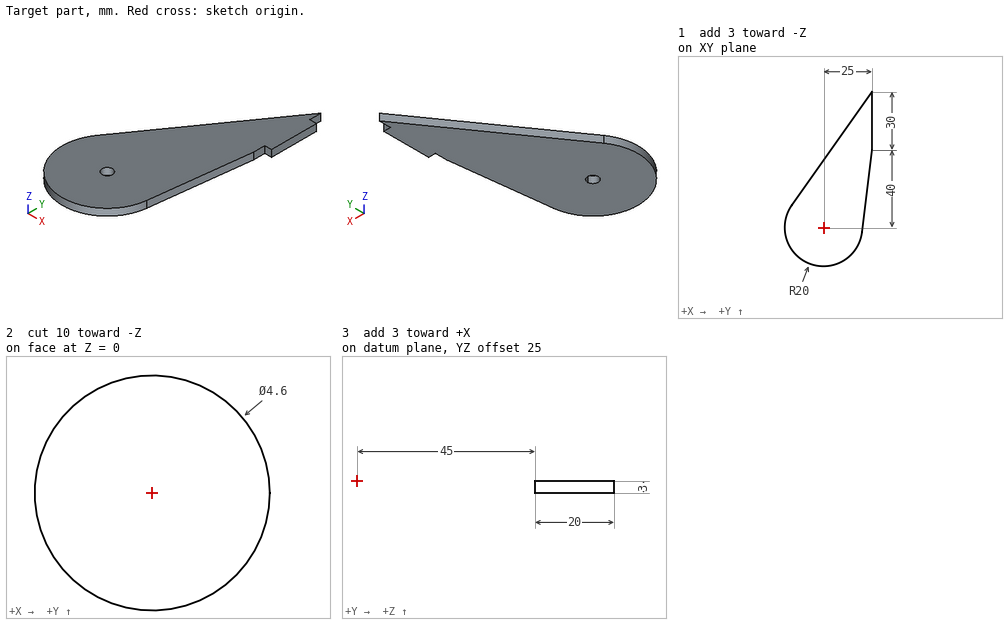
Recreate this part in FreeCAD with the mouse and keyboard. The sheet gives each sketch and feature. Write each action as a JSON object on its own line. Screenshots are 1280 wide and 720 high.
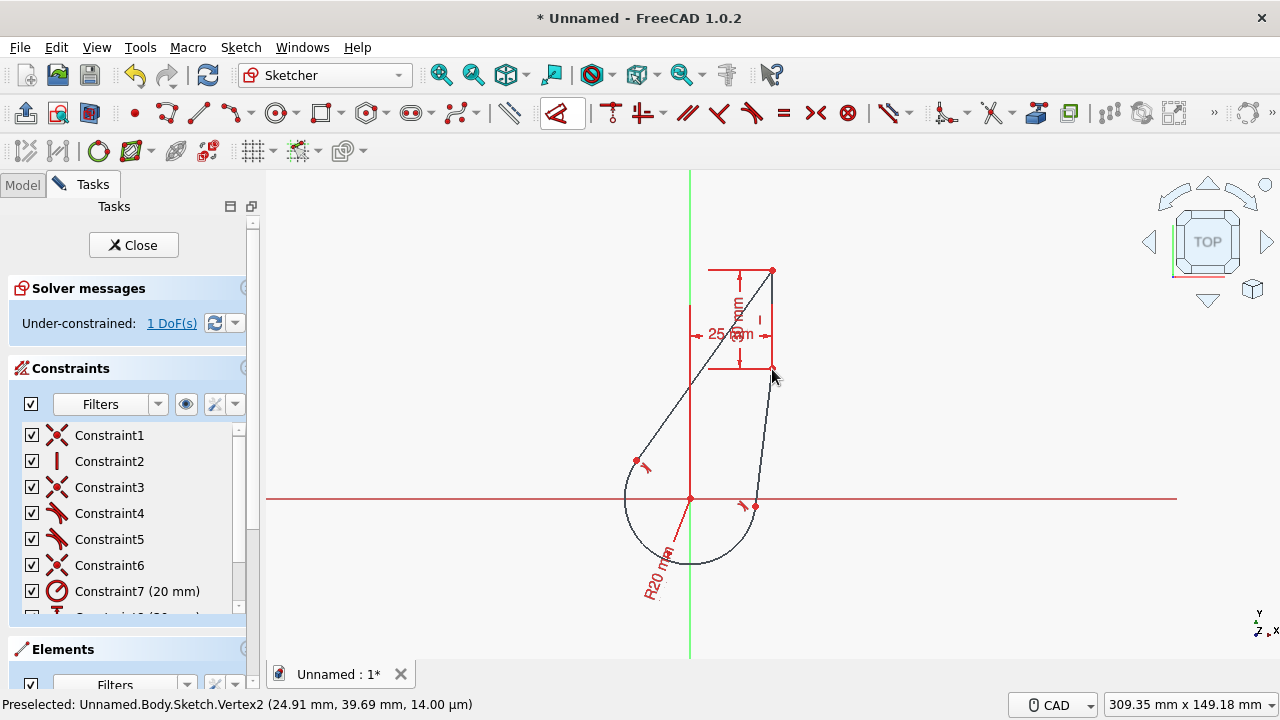
{"action": "left_click", "coordinate": [772, 369]}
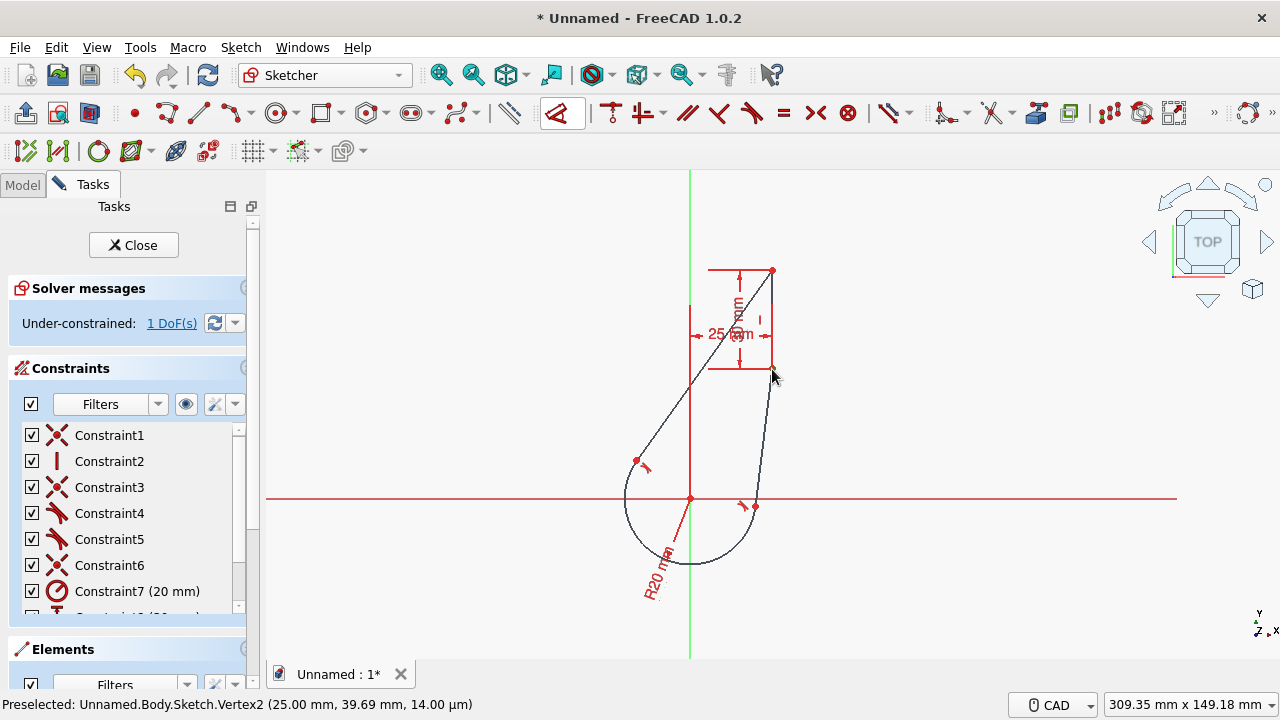
{"action": "key", "text": "i"}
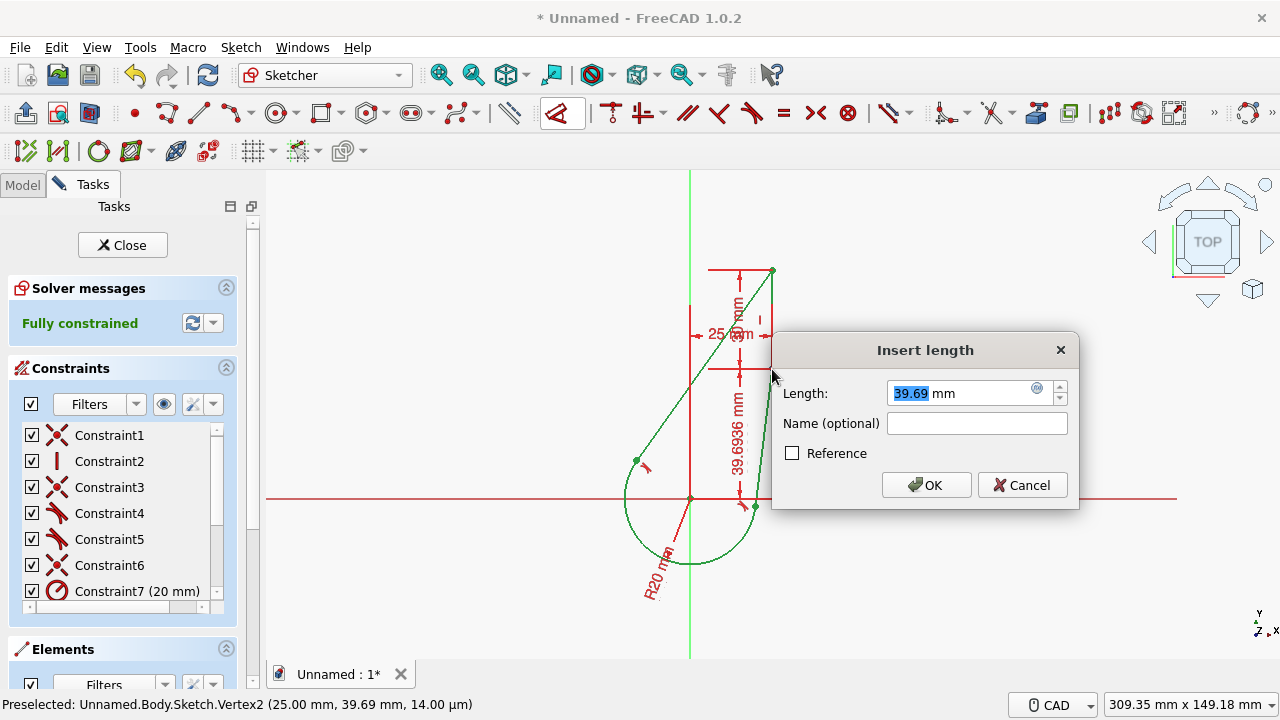
{"action": "type", "text": "40"}
{"action": "key", "text": "Return"}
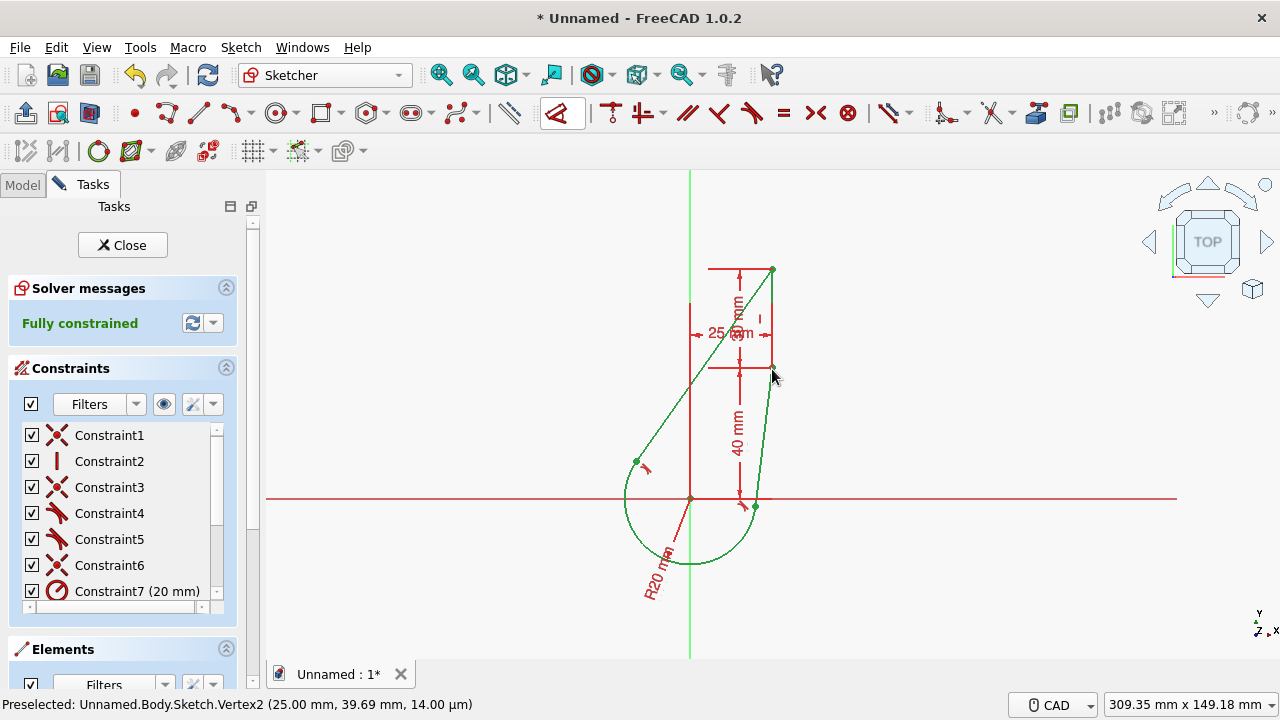
{"action": "left_click", "coordinate": [123, 245]}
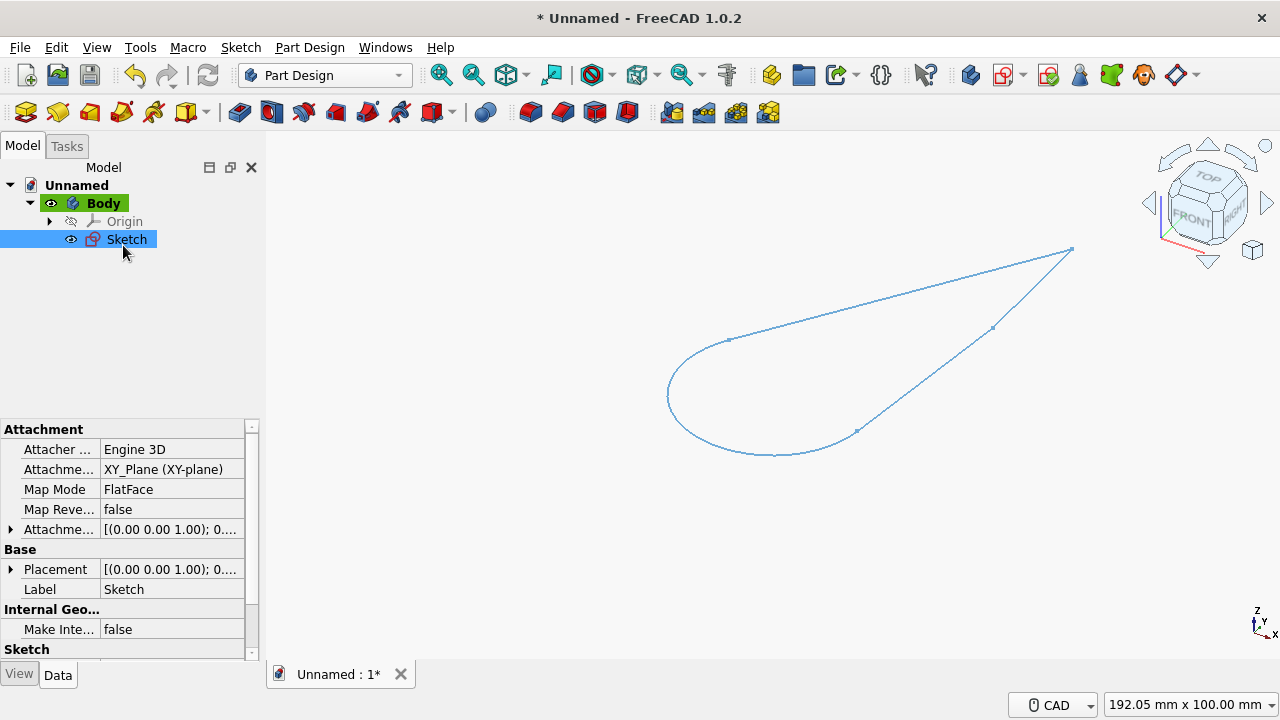
{"action": "left_click", "coordinate": [26, 112]}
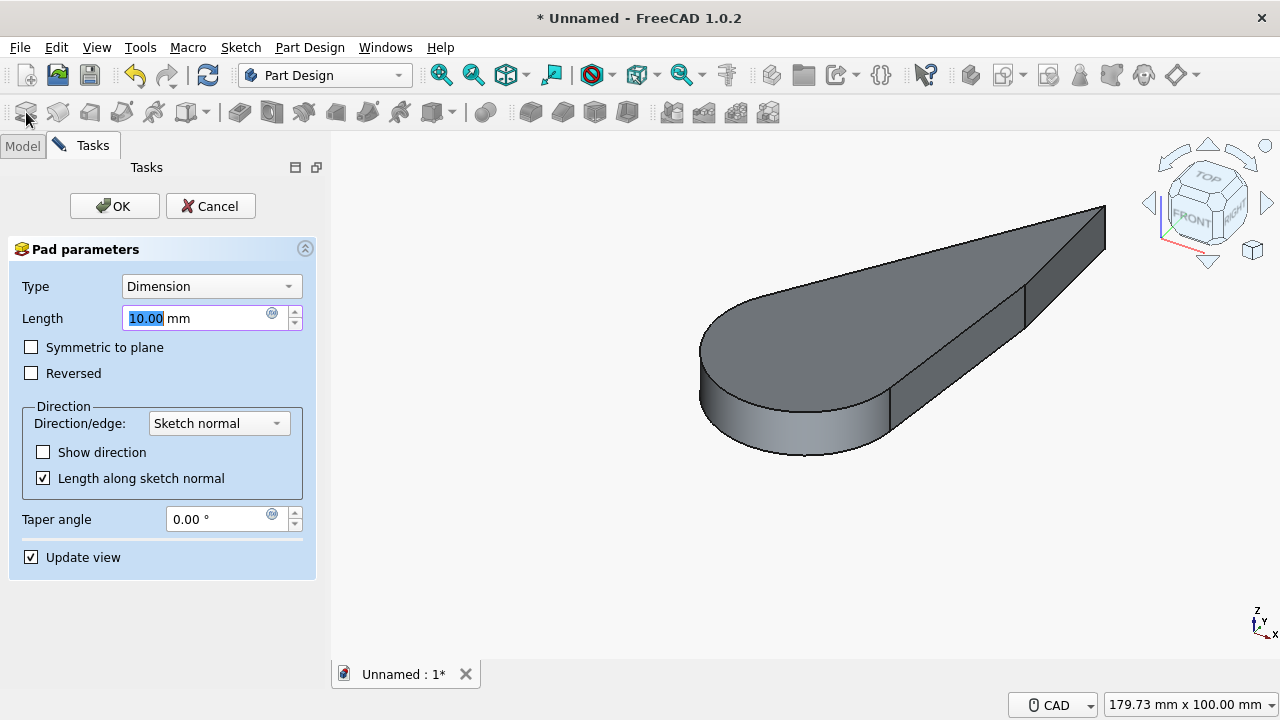
{"action": "type", "text": "3"}
{"action": "key", "text": "Tab"}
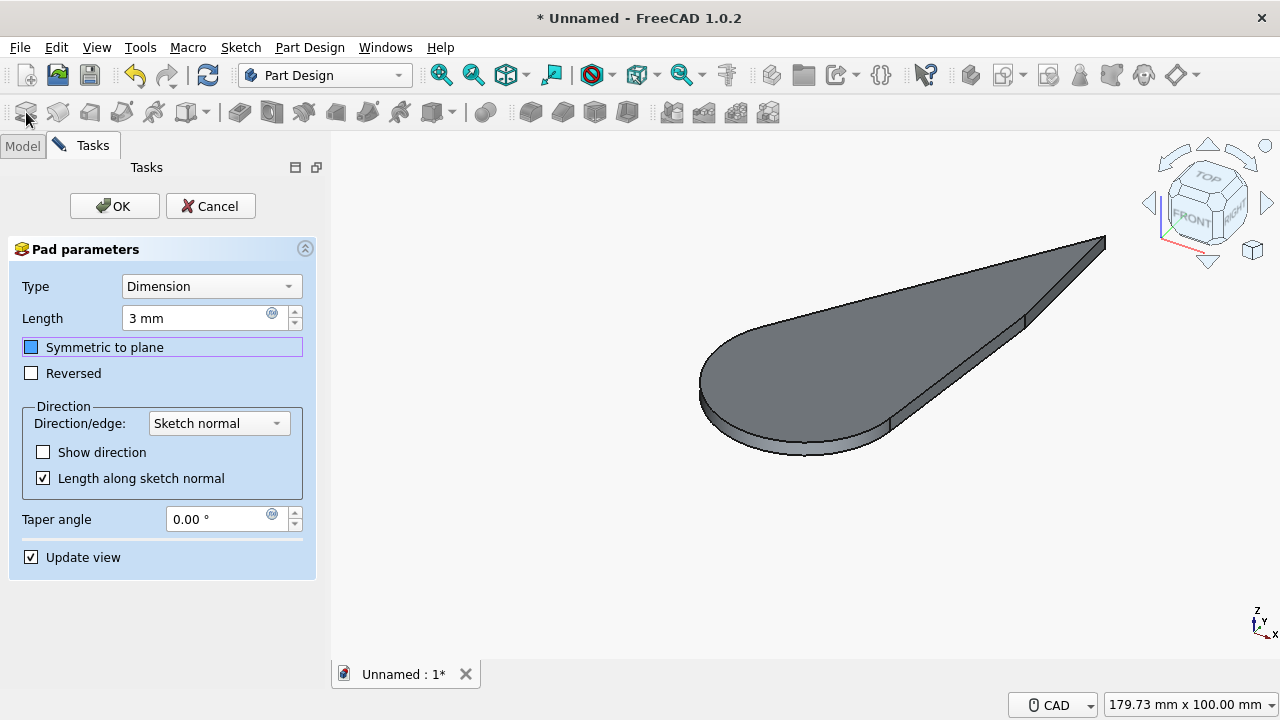
{"action": "left_click", "coordinate": [30, 373]}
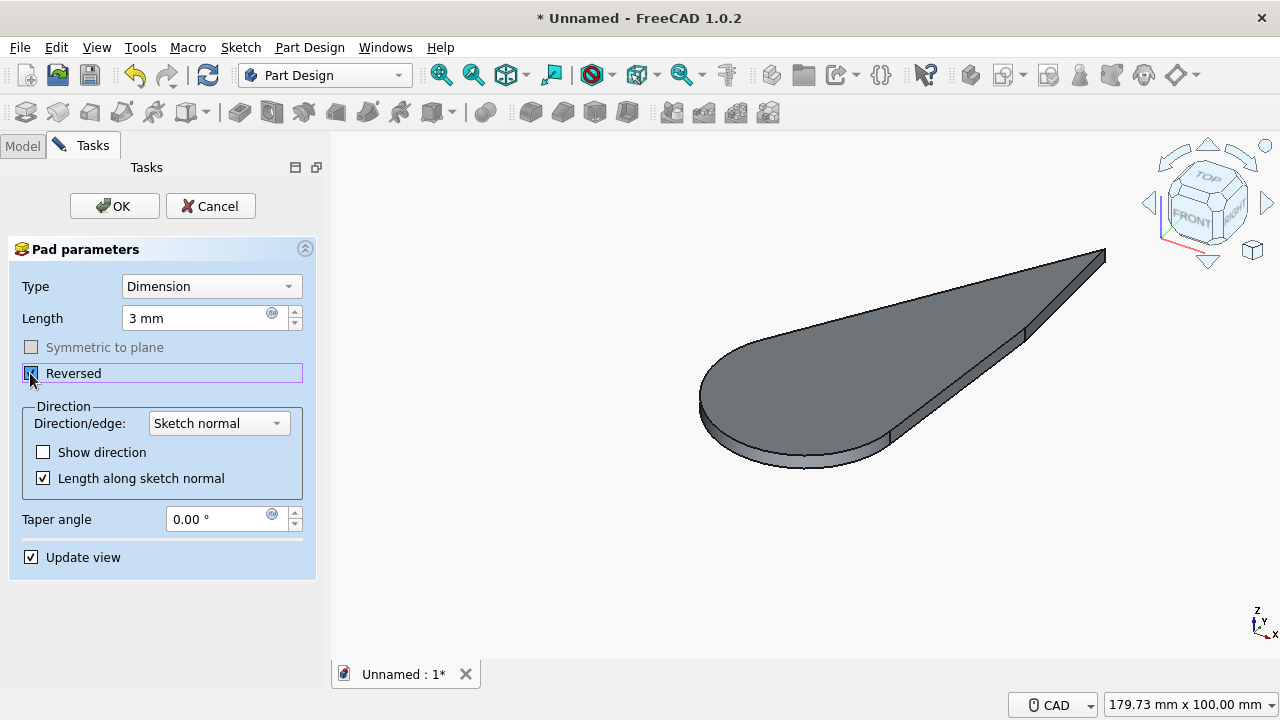
{"action": "left_click", "coordinate": [115, 206]}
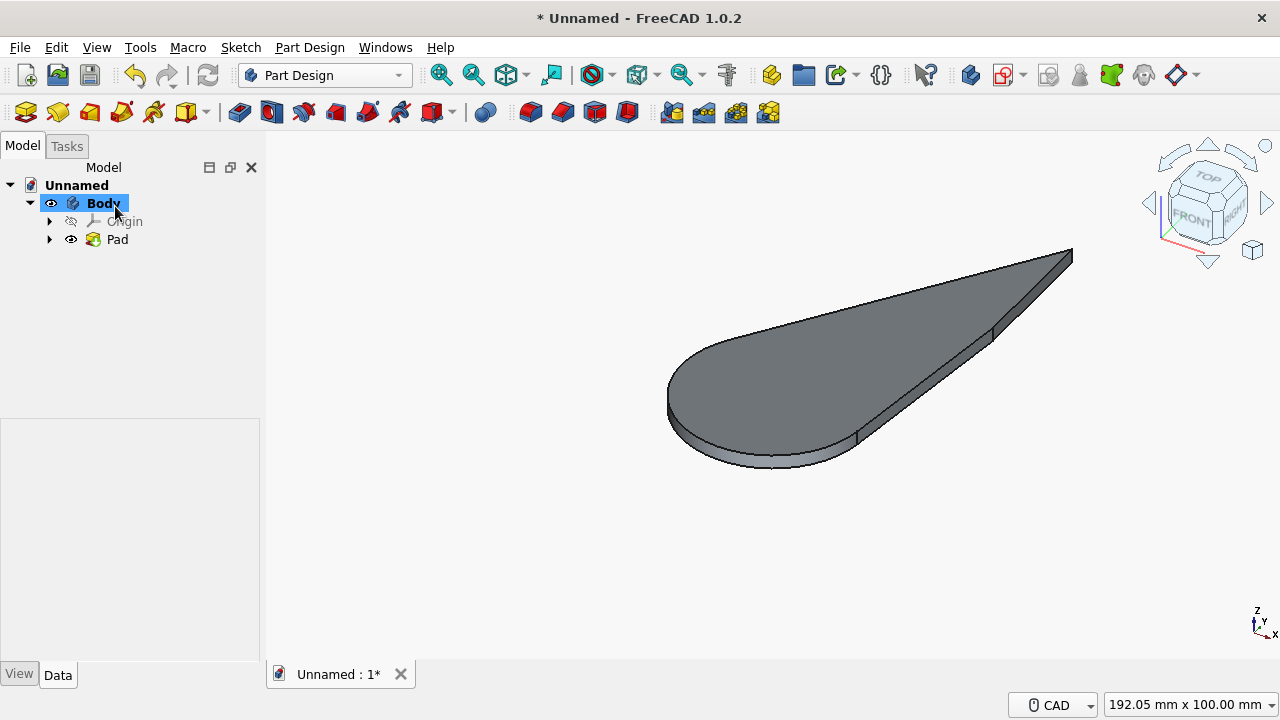
{"action": "left_click", "coordinate": [783, 400]}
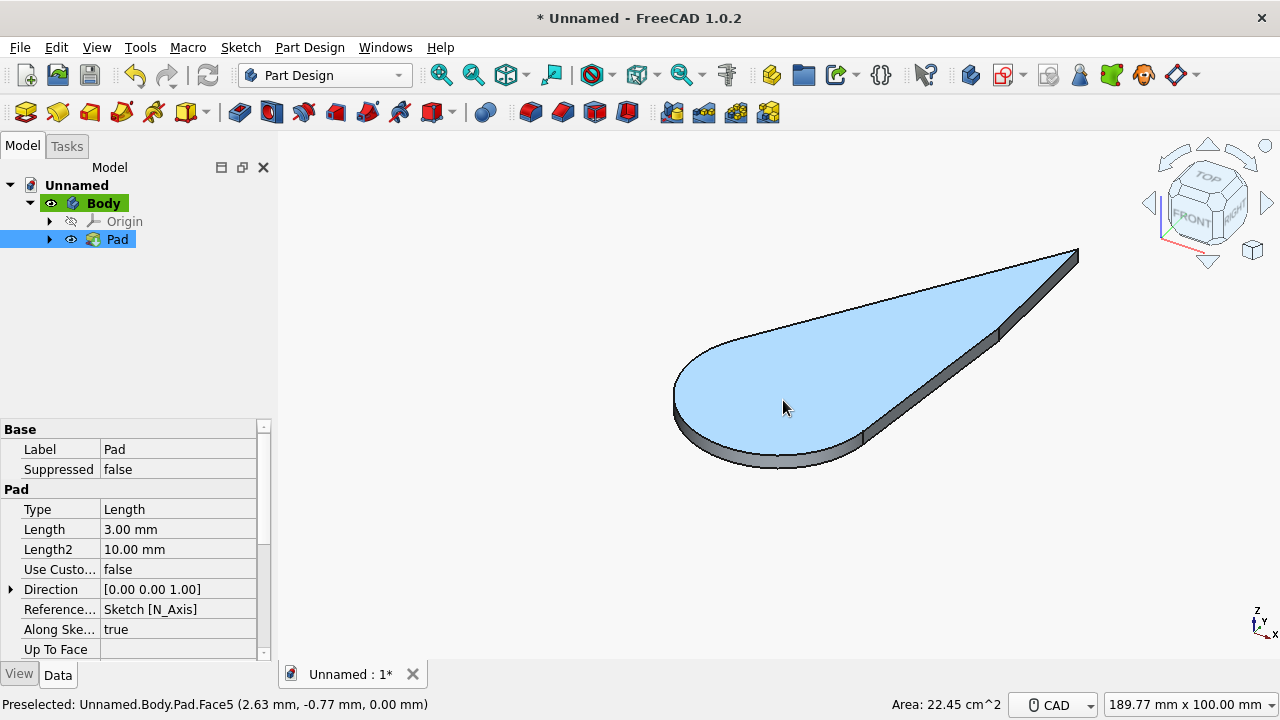
{"action": "left_click", "coordinate": [1004, 76]}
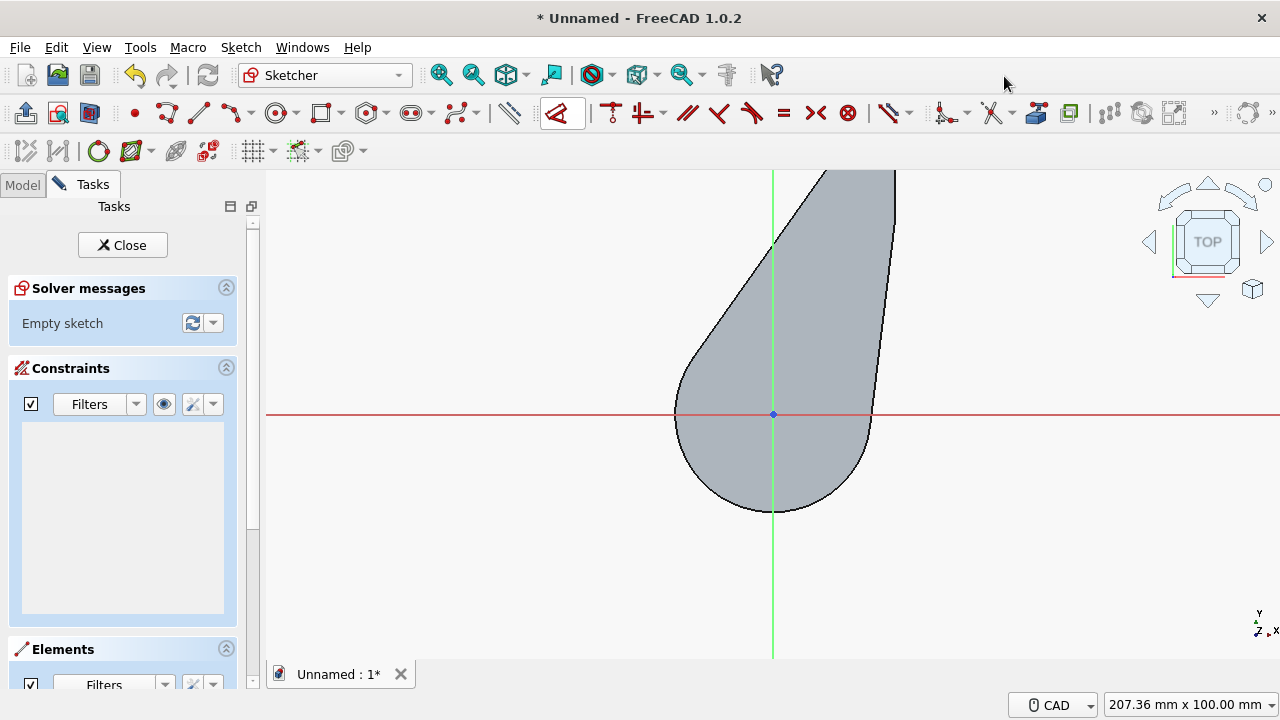
{"action": "scroll", "coordinate": [778, 415], "scroll_direction": "up", "scroll_amount": 13}